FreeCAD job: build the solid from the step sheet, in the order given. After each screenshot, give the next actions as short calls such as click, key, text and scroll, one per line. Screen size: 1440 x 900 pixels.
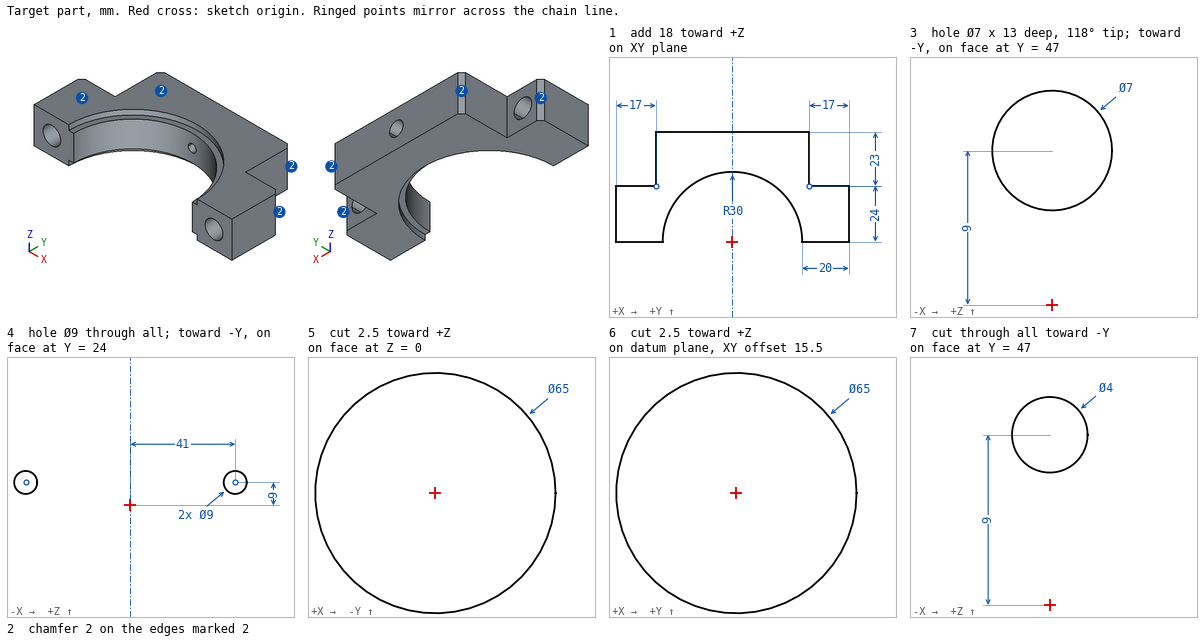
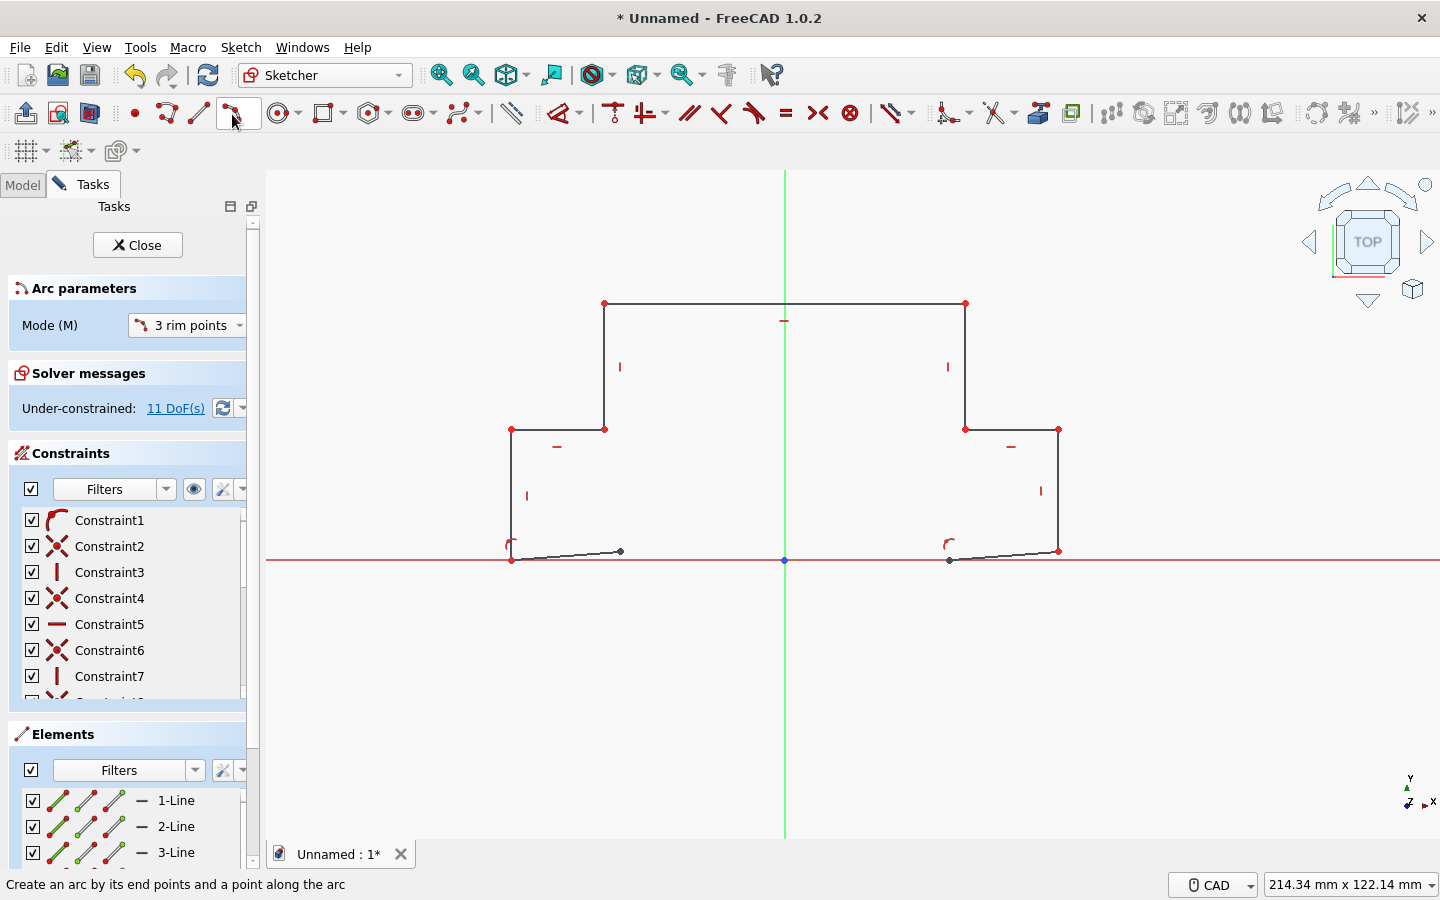
click(620, 552)
click(949, 560)
click(835, 404)
key(Escape)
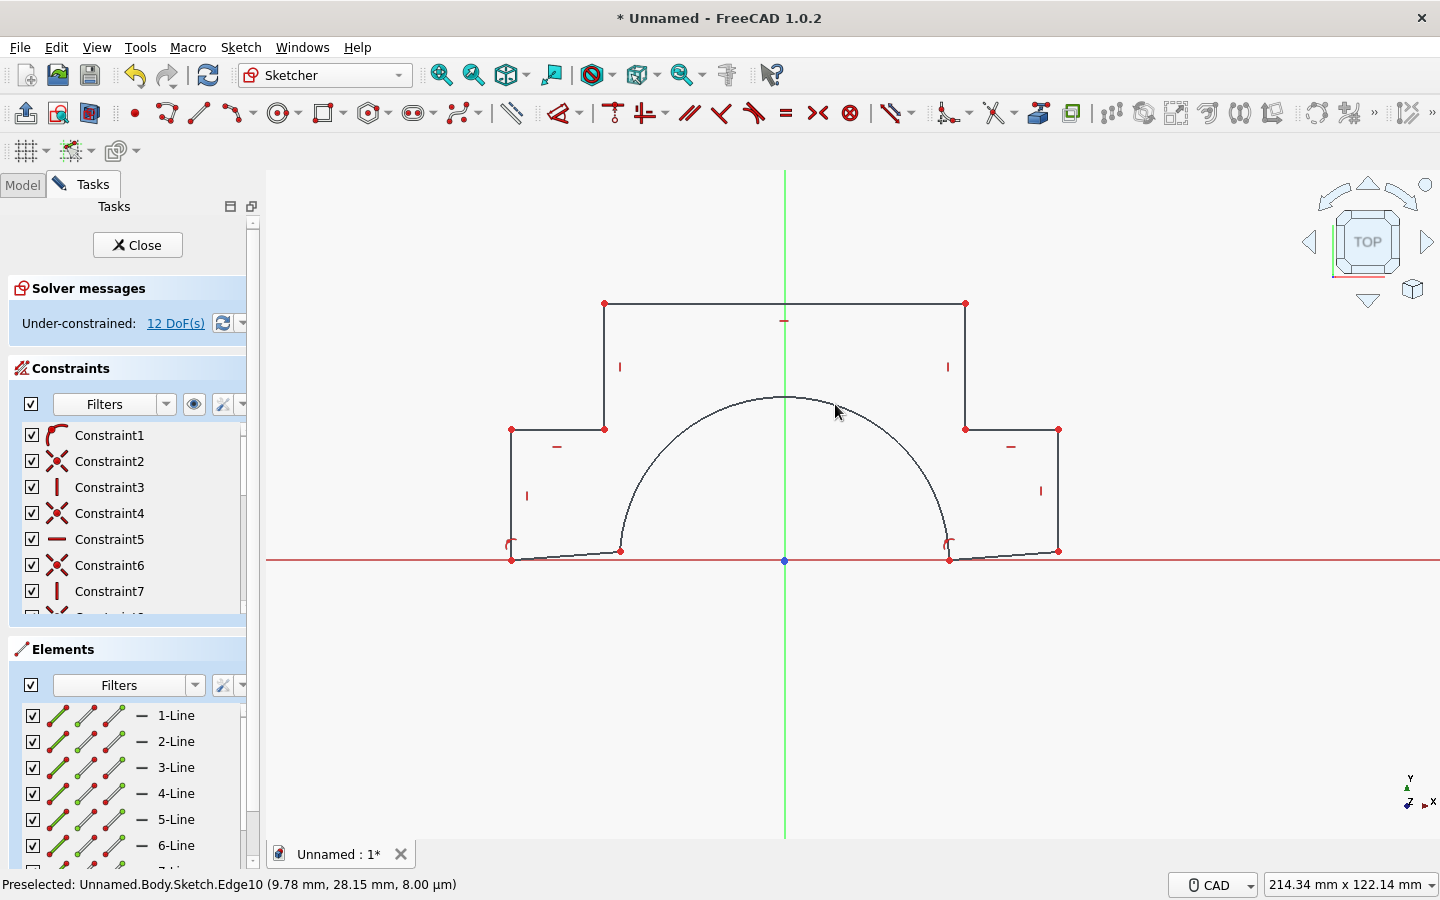
click(982, 558)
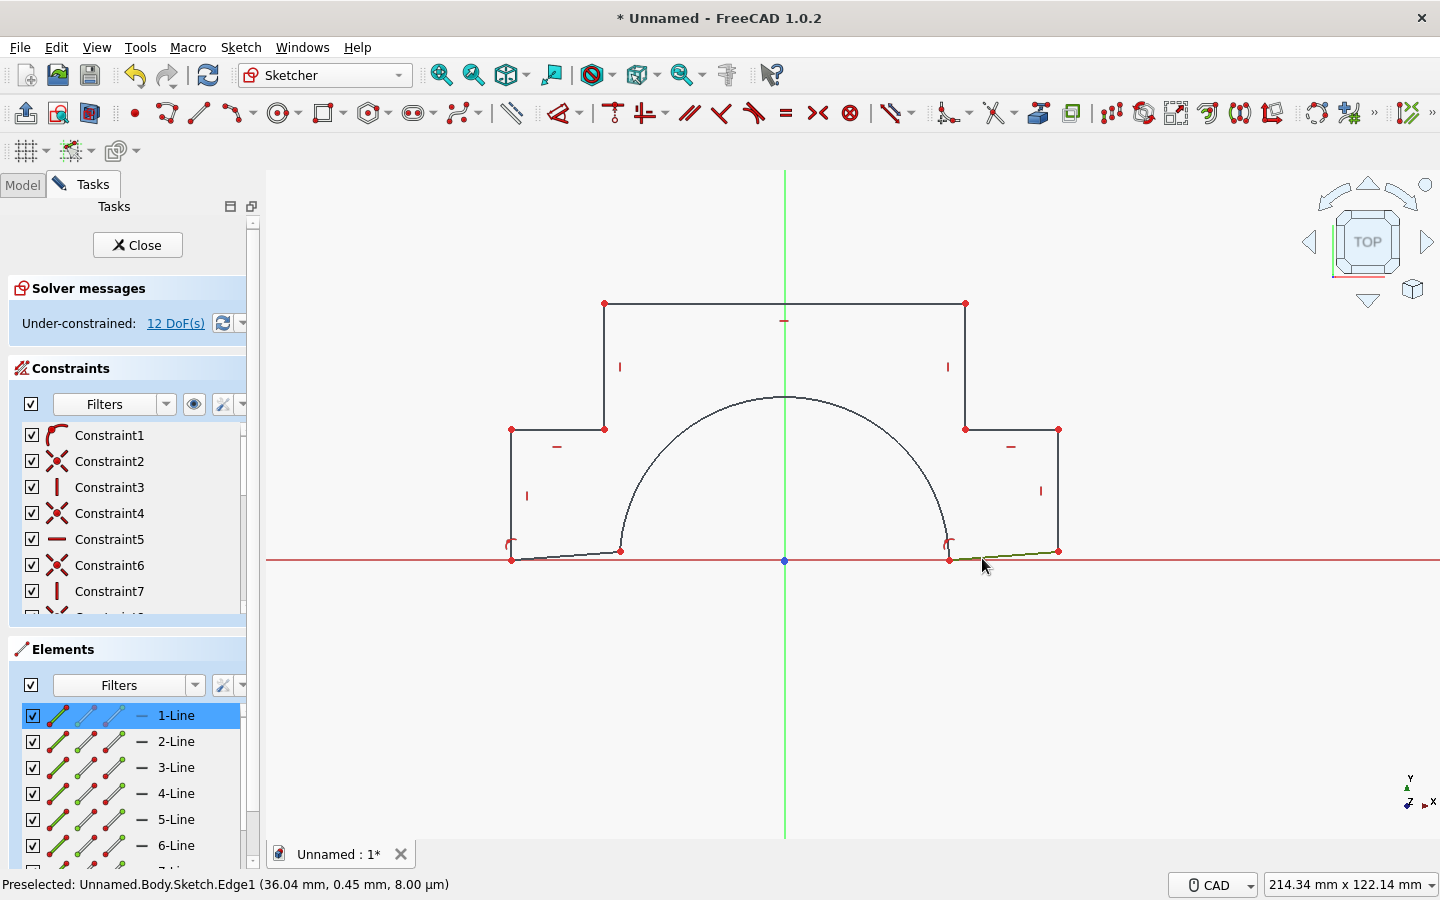
click(668, 114)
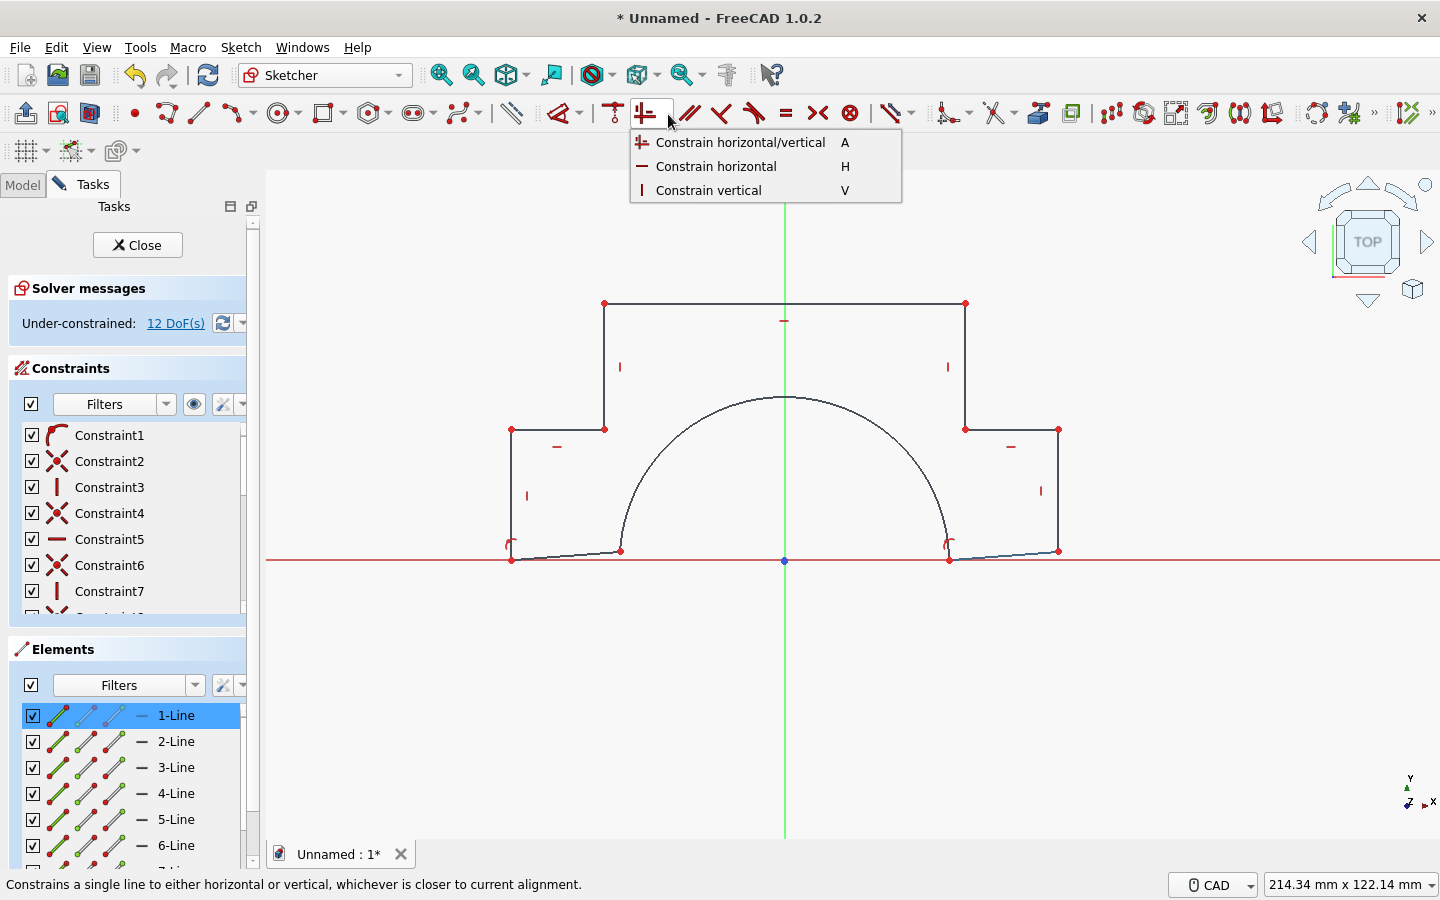
click(766, 166)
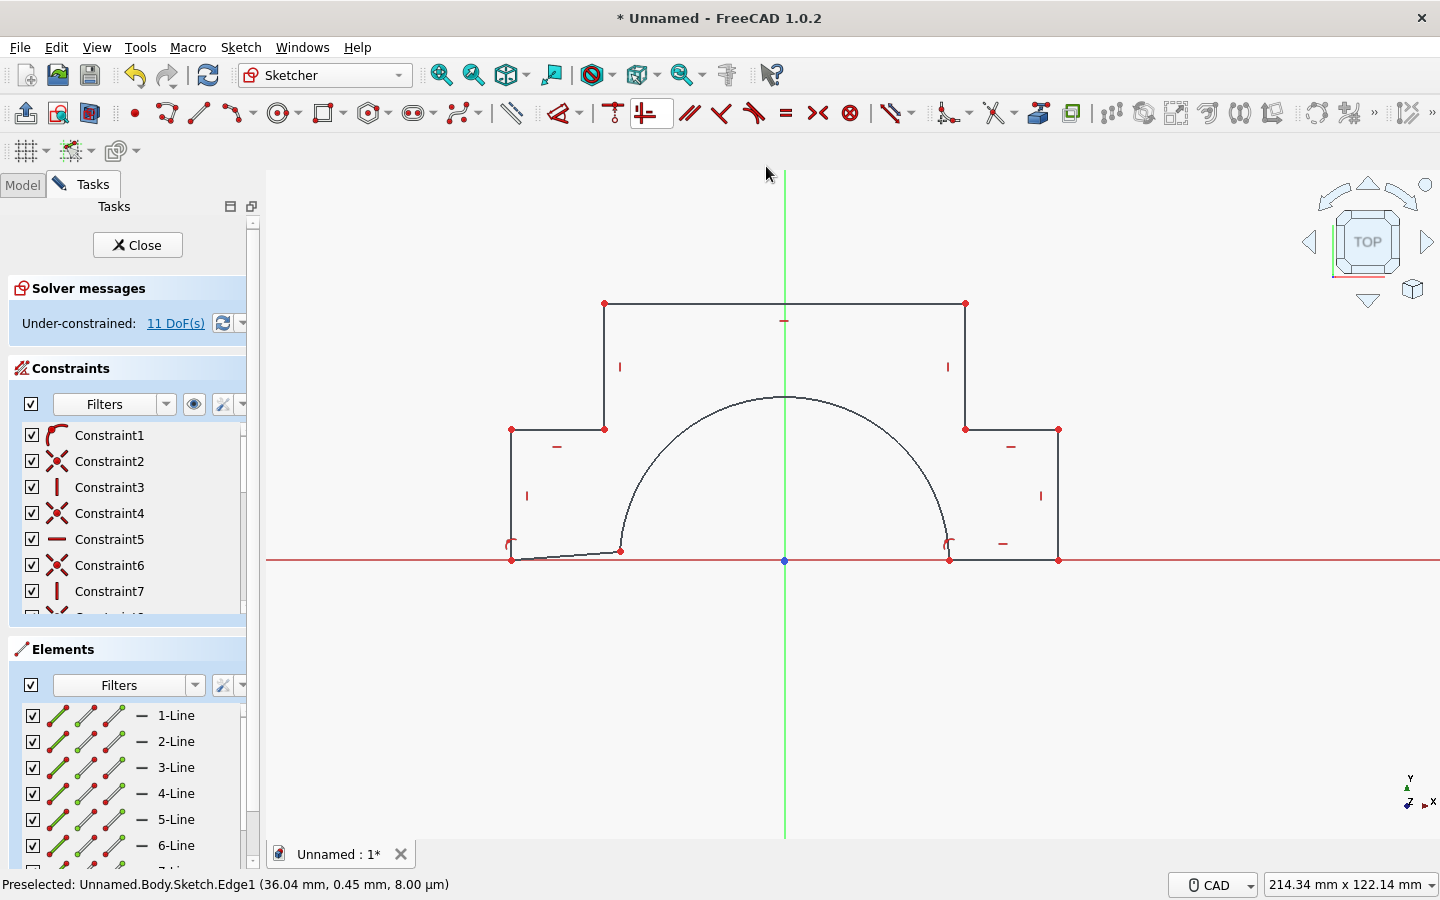
click(544, 558)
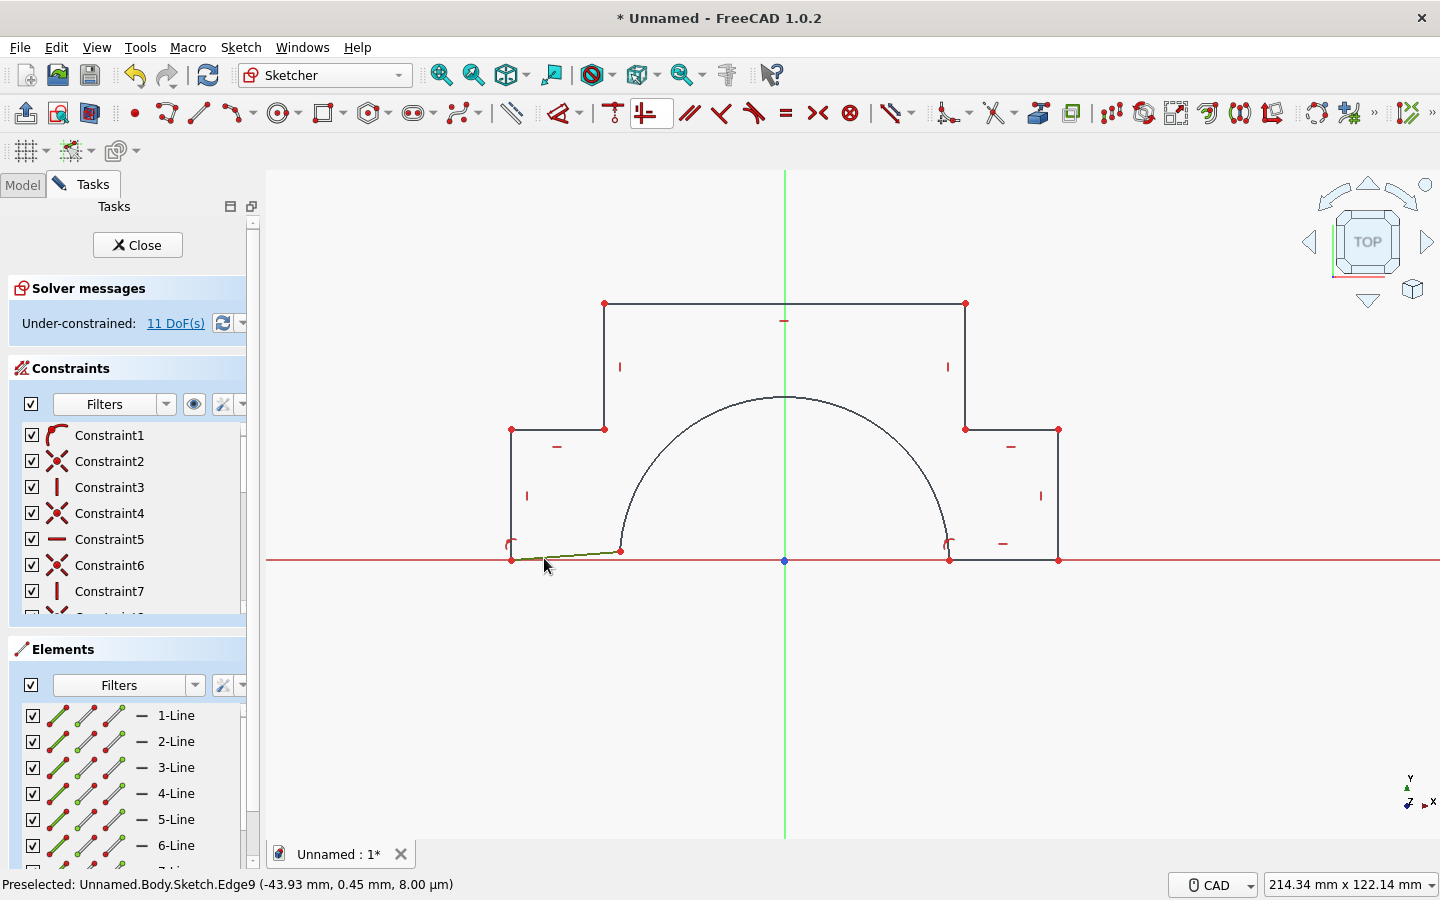
key(h)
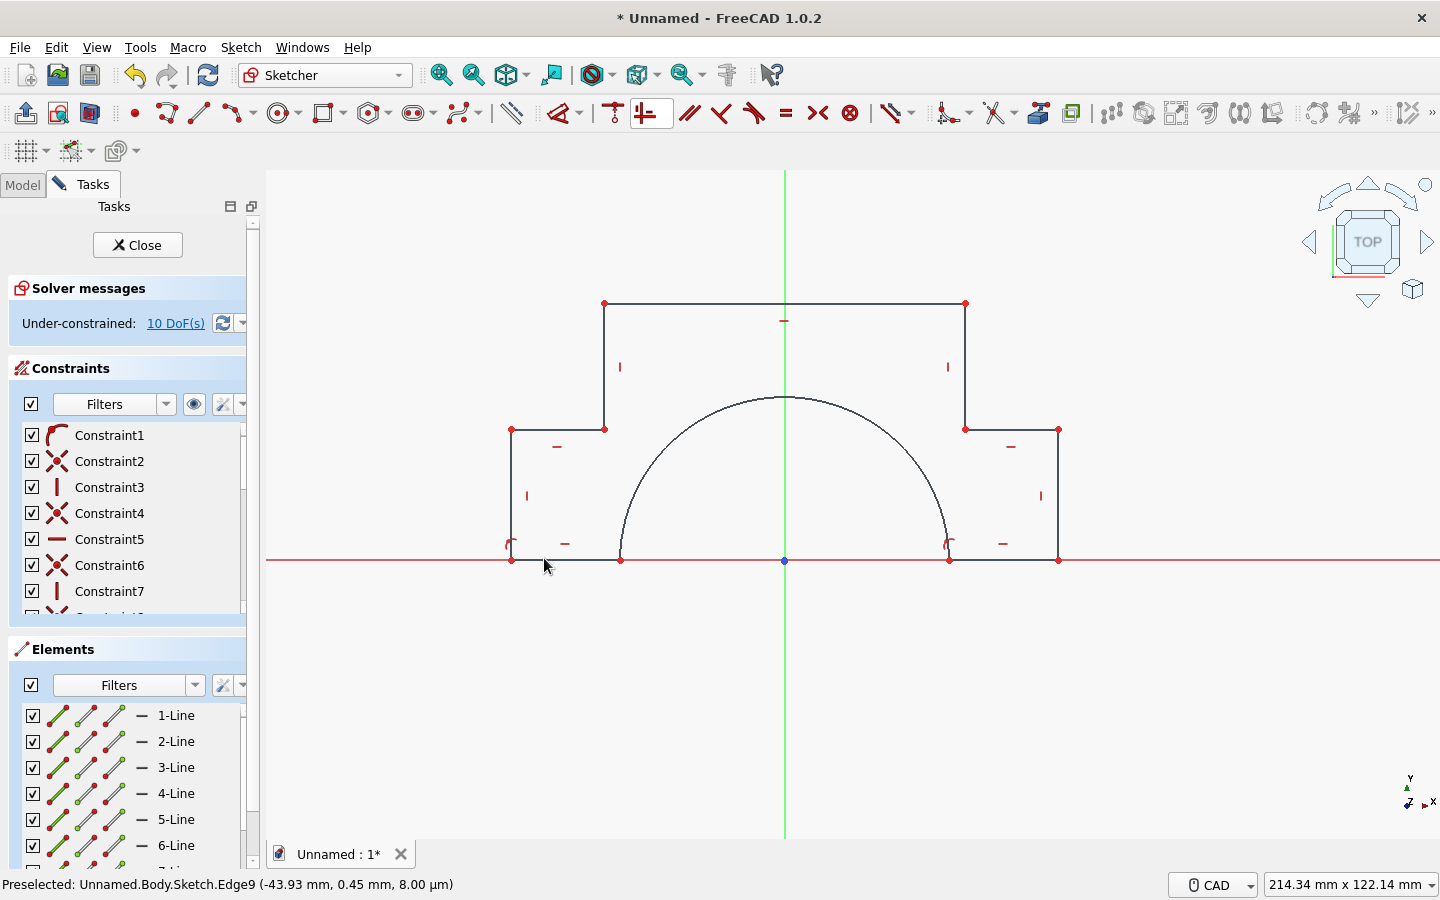
drag(774, 550, 795, 572)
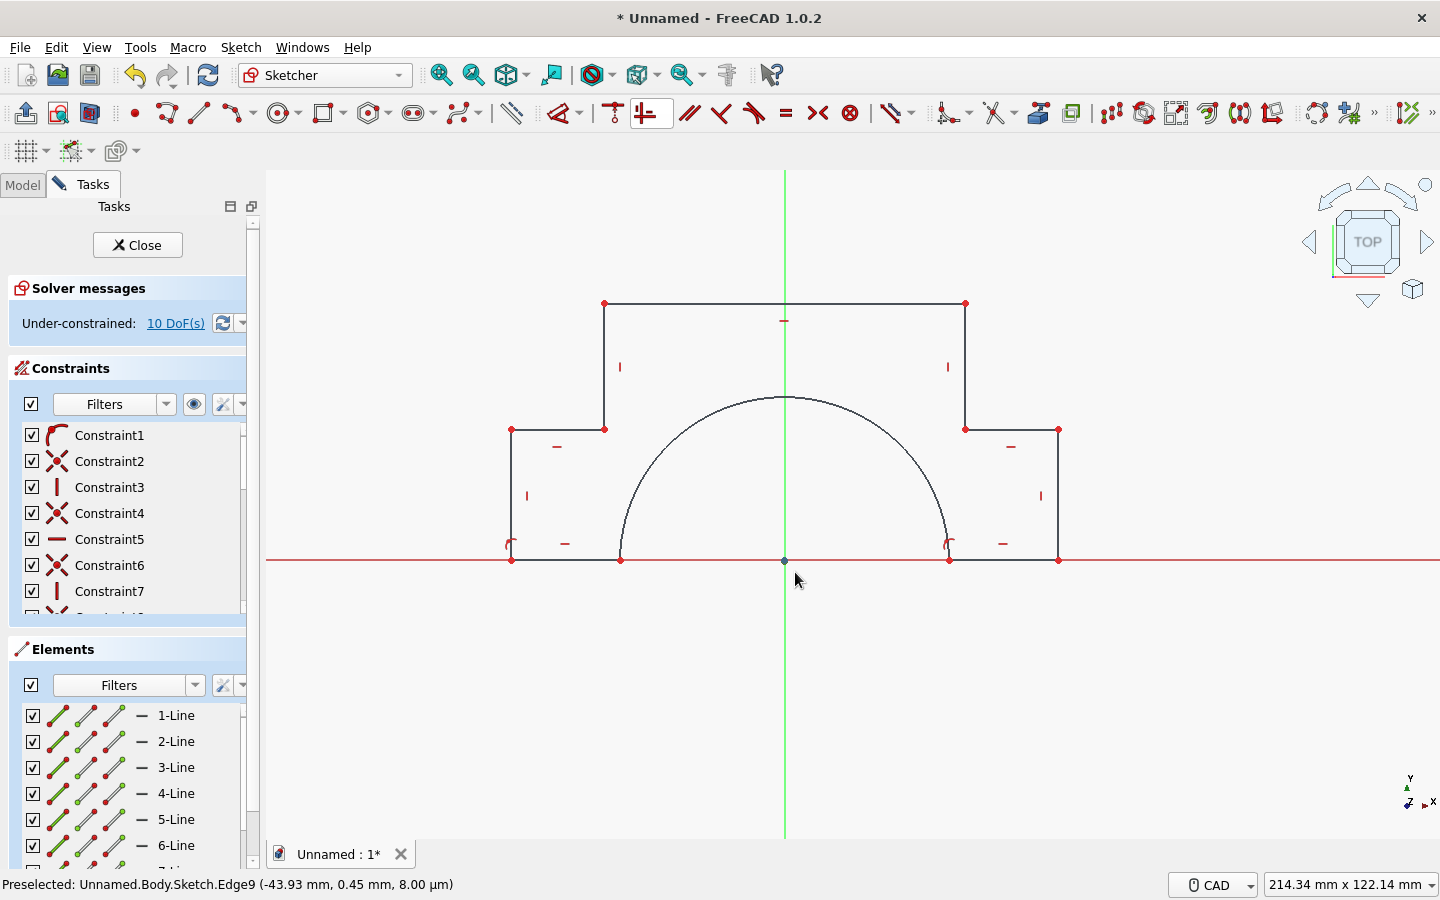
click(614, 114)